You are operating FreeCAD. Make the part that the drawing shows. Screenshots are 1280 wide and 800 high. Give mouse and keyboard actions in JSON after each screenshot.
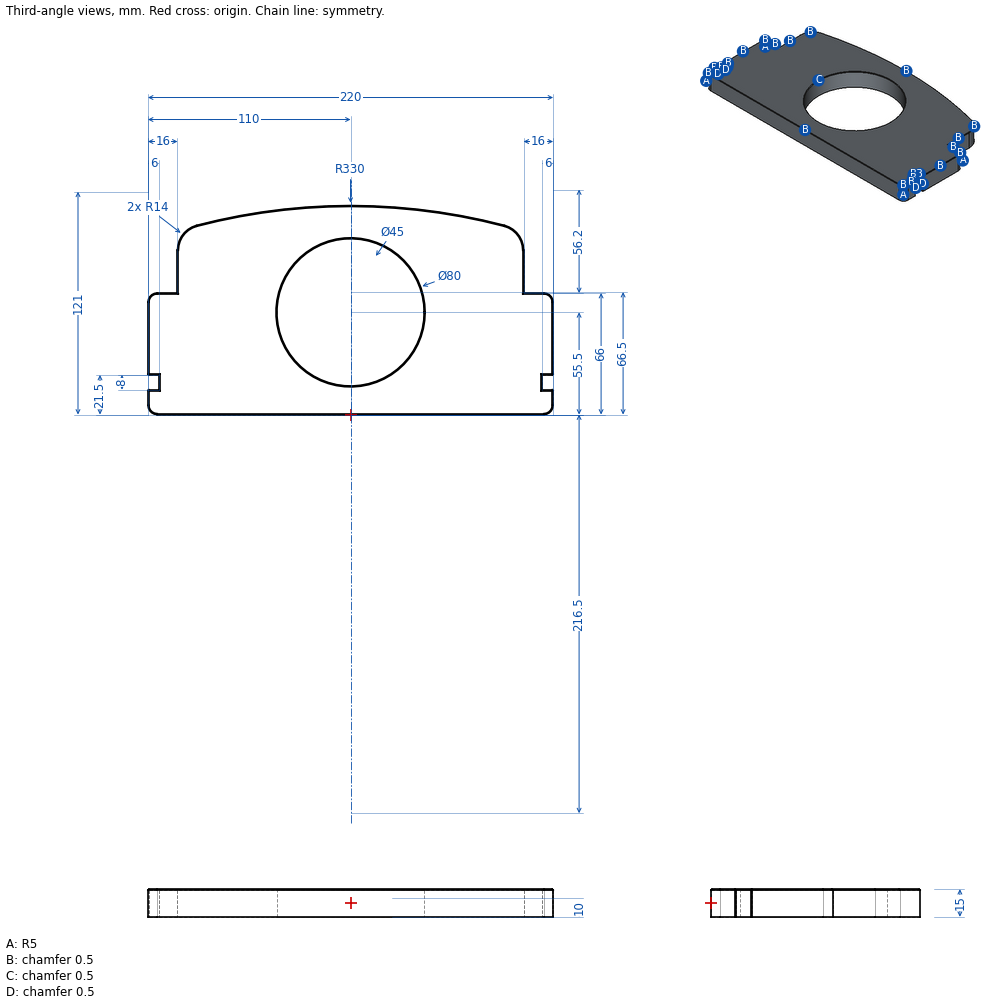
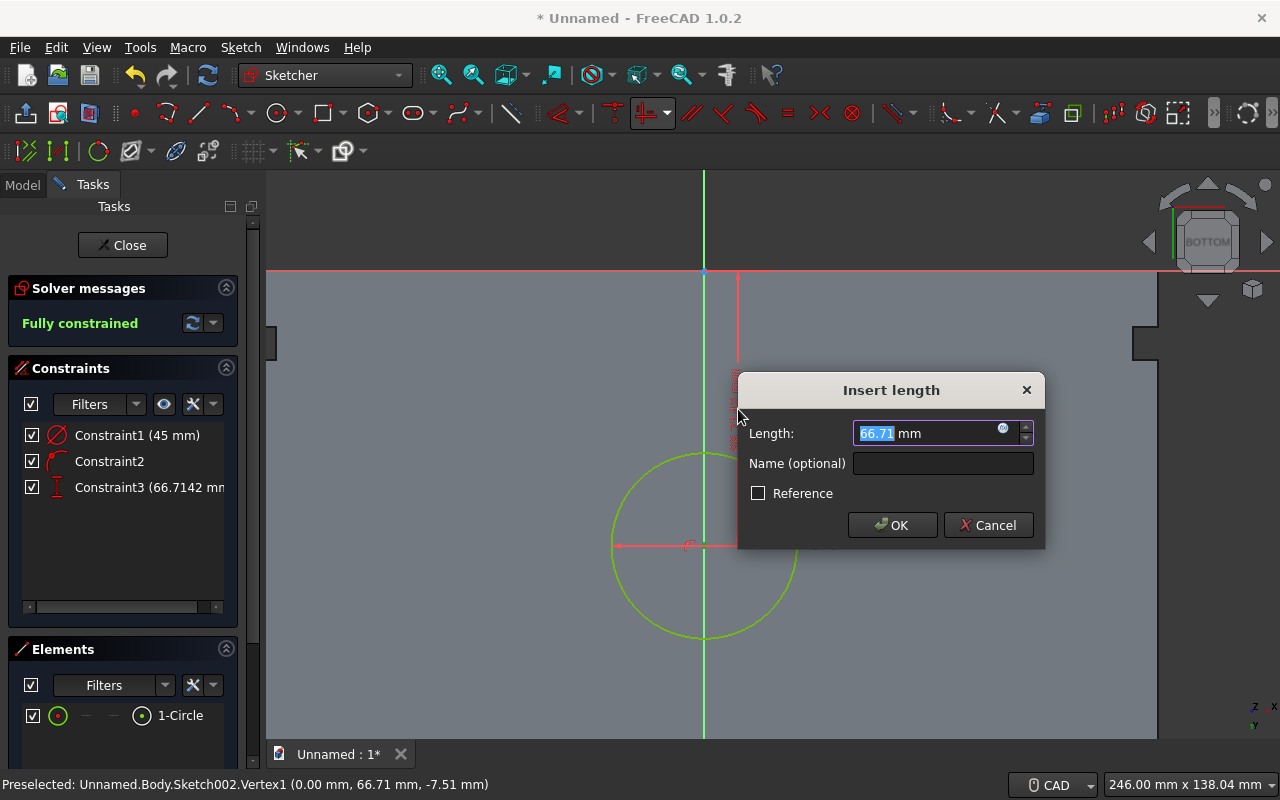
{"action": "type", "text": "66.5"}
{"action": "key", "text": "Return"}
{"action": "key", "text": "Escape"}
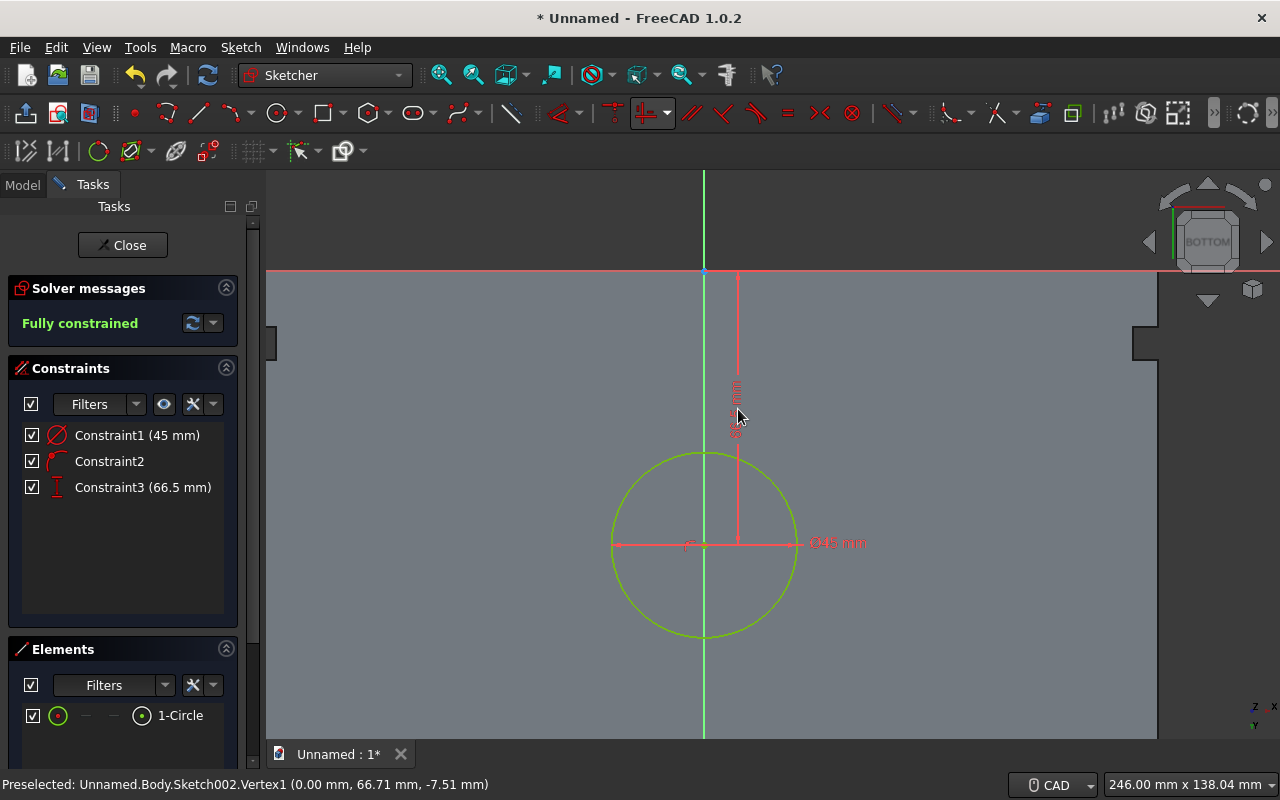
{"action": "left_click", "coordinate": [123, 245]}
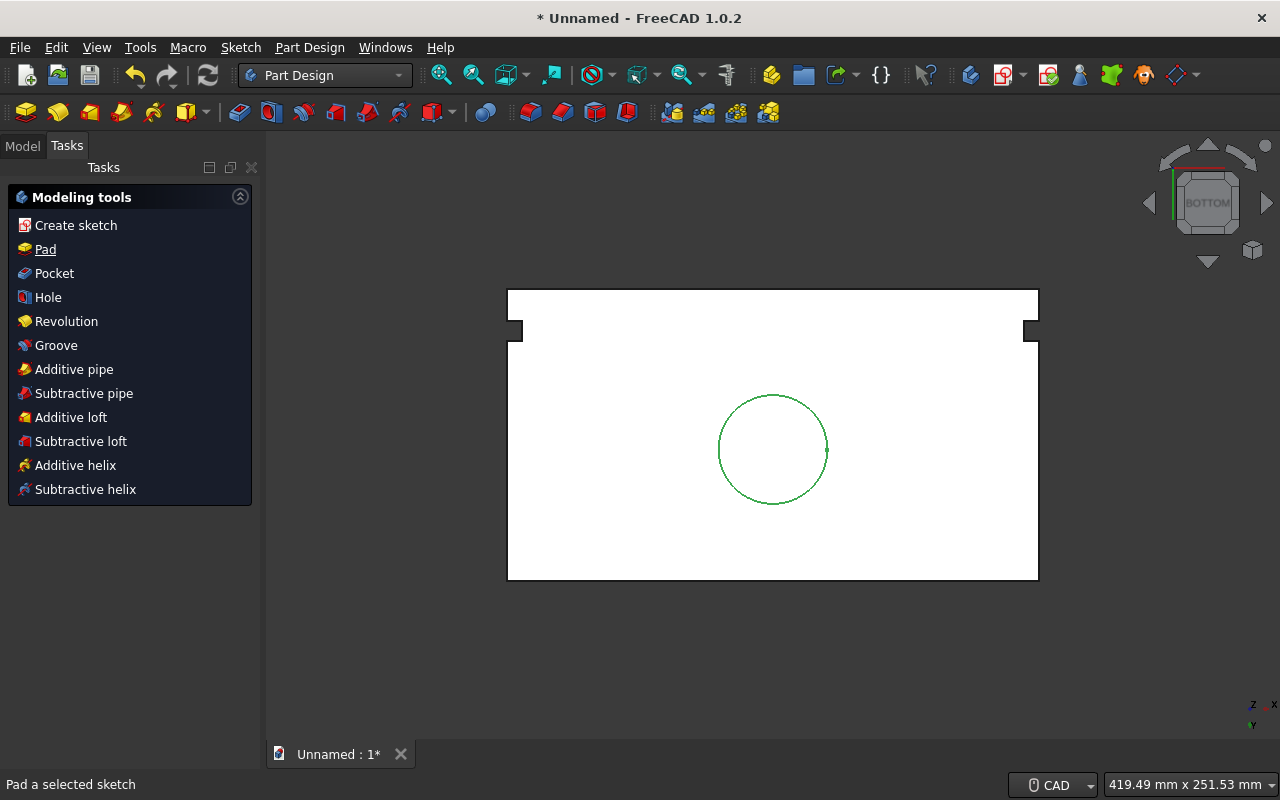
{"action": "left_click", "coordinate": [240, 112]}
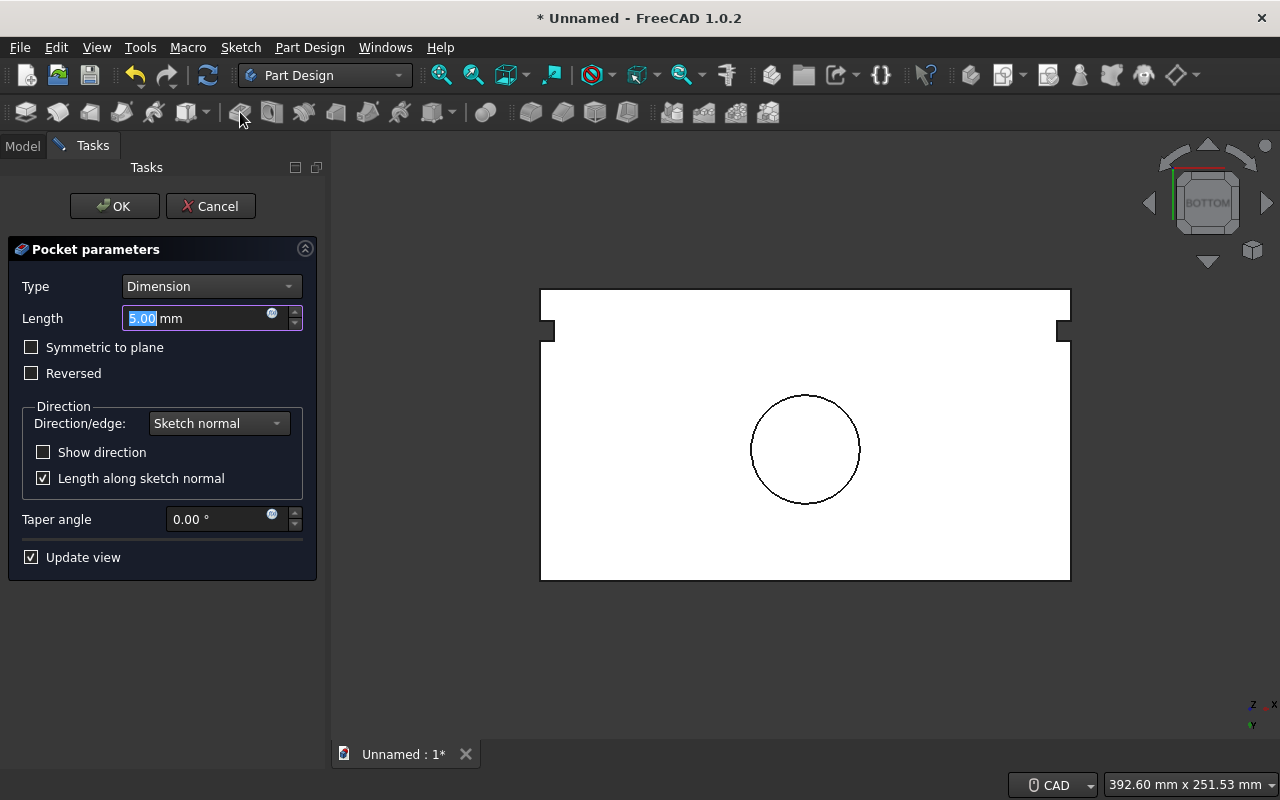
{"action": "type", "text": "10"}
{"action": "key", "text": "Tab"}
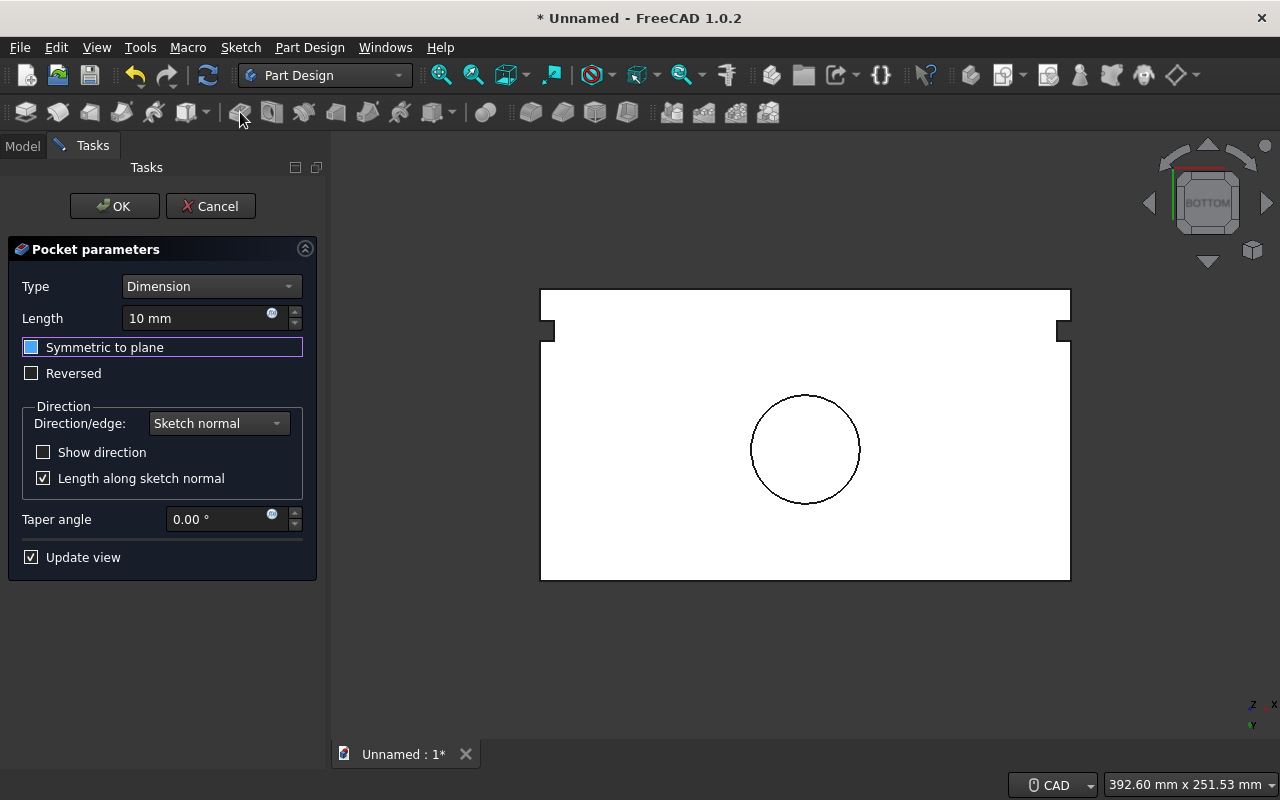
{"action": "left_click", "coordinate": [115, 206]}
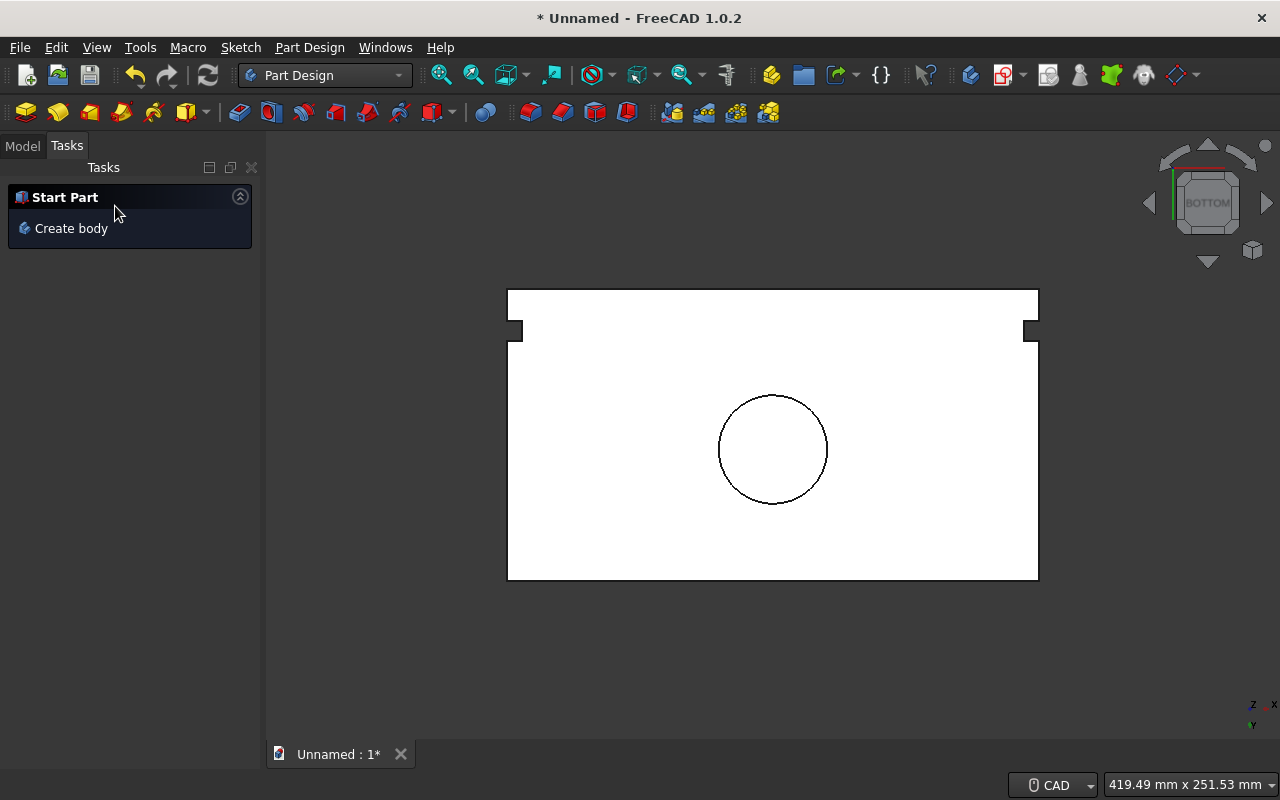
{"action": "key", "text": "0"}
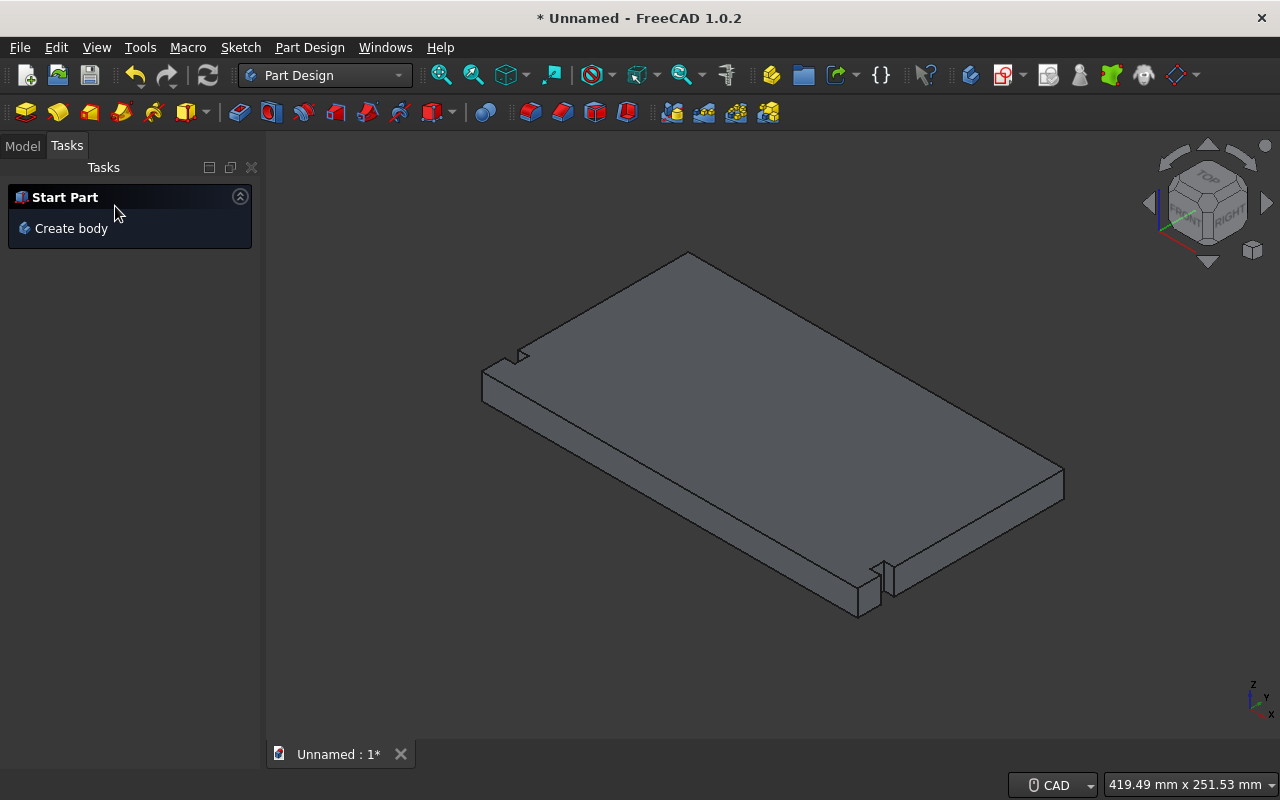
{"action": "left_click", "coordinate": [827, 450]}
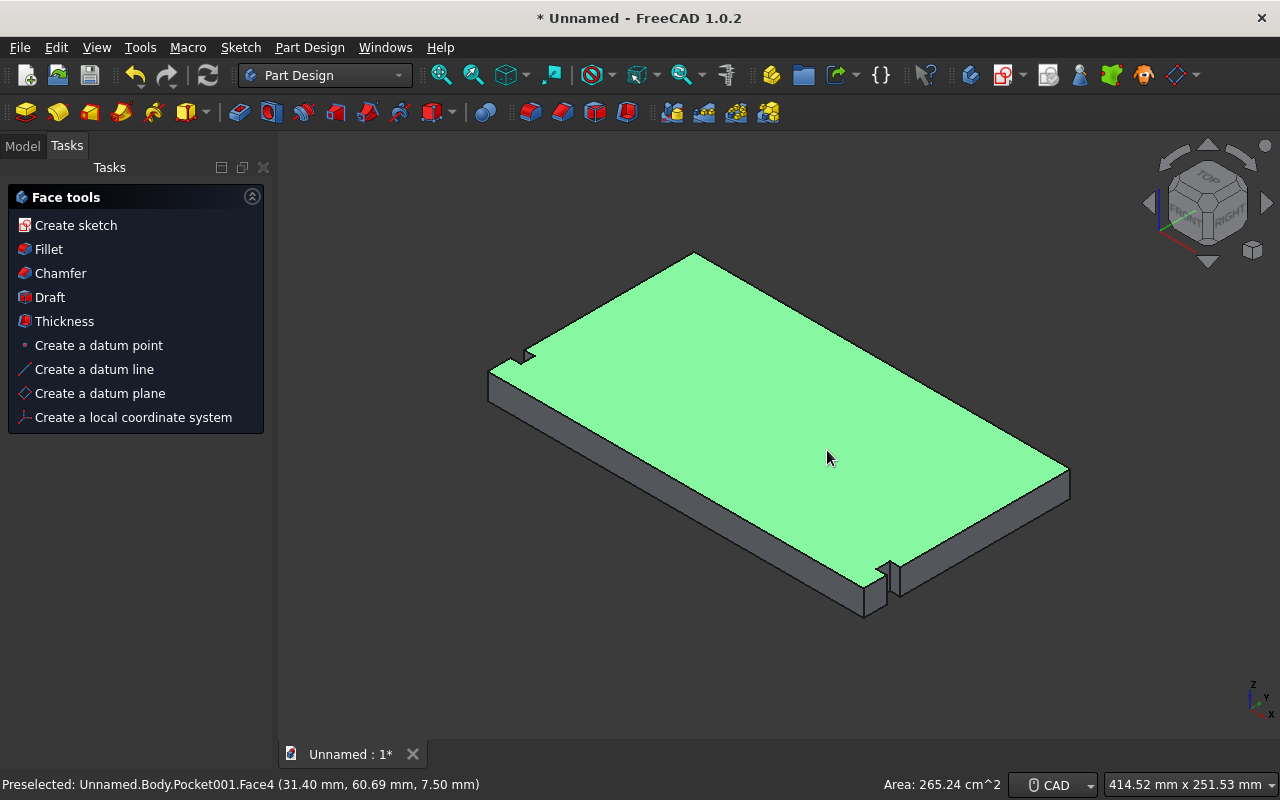
{"action": "left_click", "coordinate": [1004, 76]}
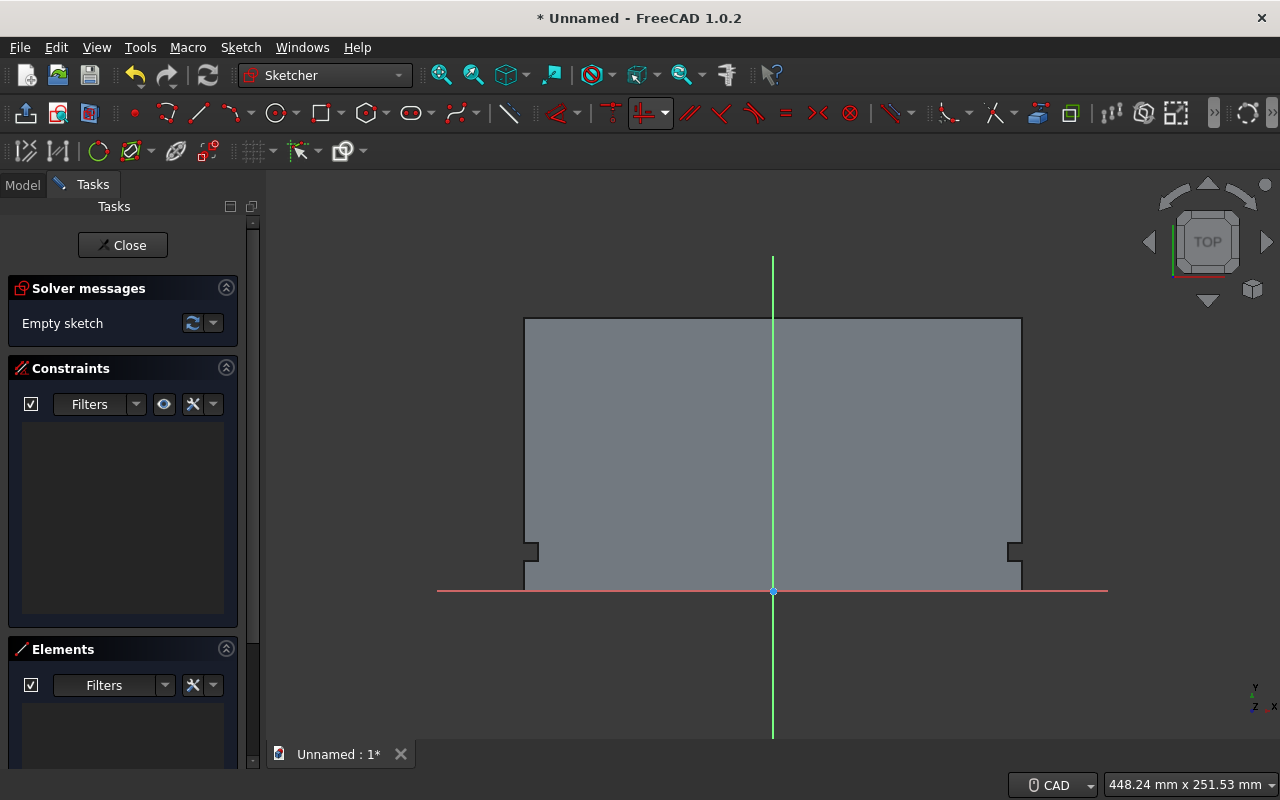
{"action": "left_click", "coordinate": [168, 114]}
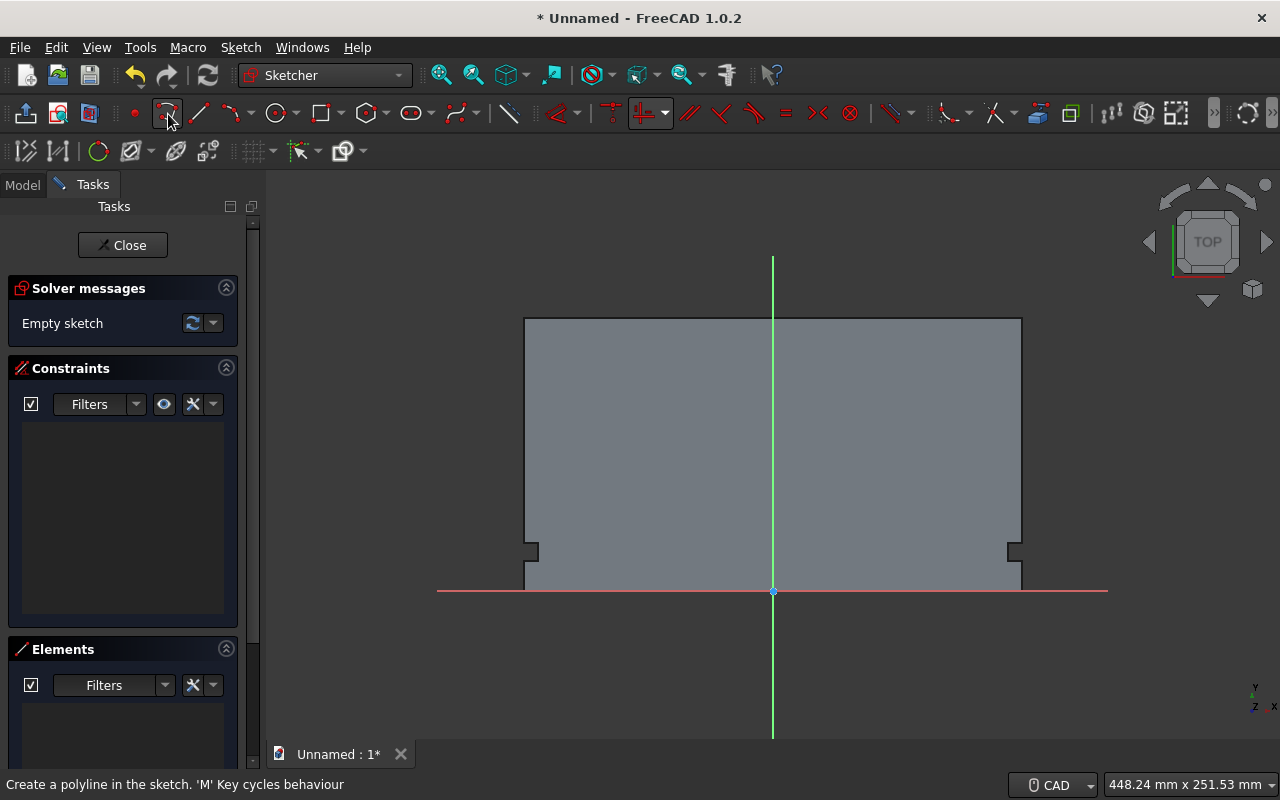
{"action": "left_click", "coordinate": [986, 390]}
{"action": "left_click", "coordinate": [986, 442]}
{"action": "left_click", "coordinate": [1022, 442]}
{"action": "left_click", "coordinate": [1022, 315]}
{"action": "left_click", "coordinate": [524, 315]}
{"action": "left_click", "coordinate": [524, 442]}
{"action": "left_click", "coordinate": [560, 442]}
{"action": "left_click", "coordinate": [560, 390]}
{"action": "right_click", "coordinate": [560, 390]}